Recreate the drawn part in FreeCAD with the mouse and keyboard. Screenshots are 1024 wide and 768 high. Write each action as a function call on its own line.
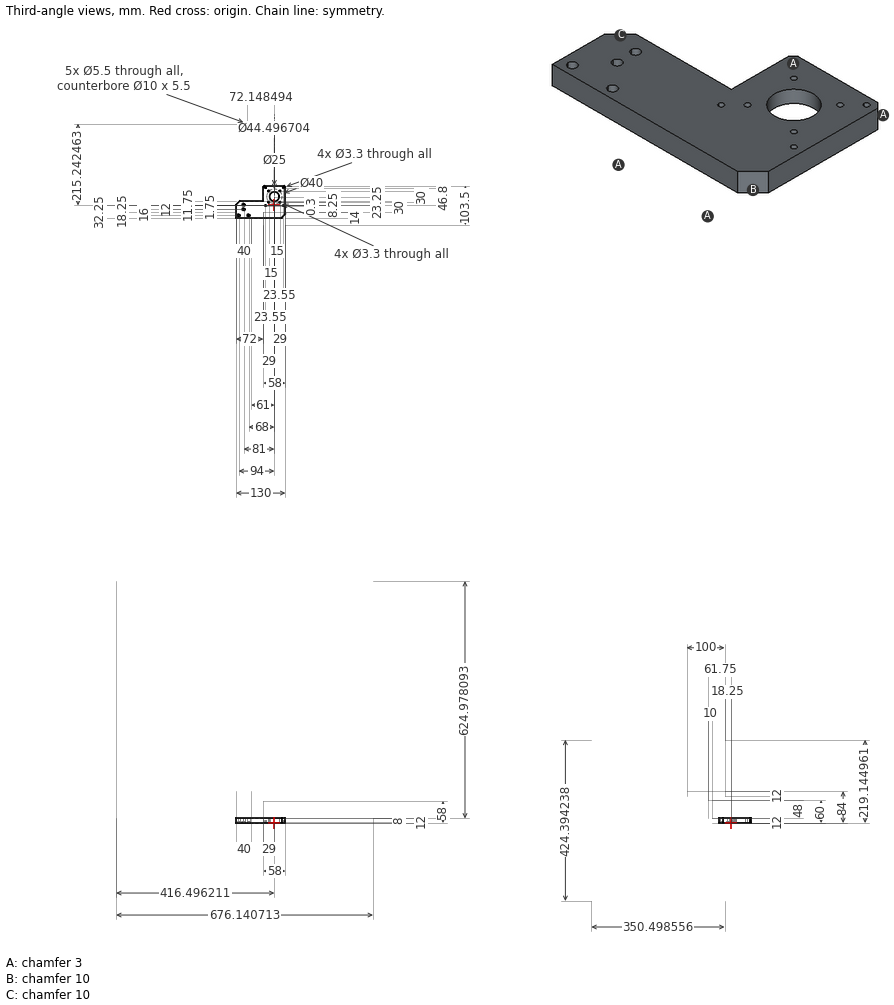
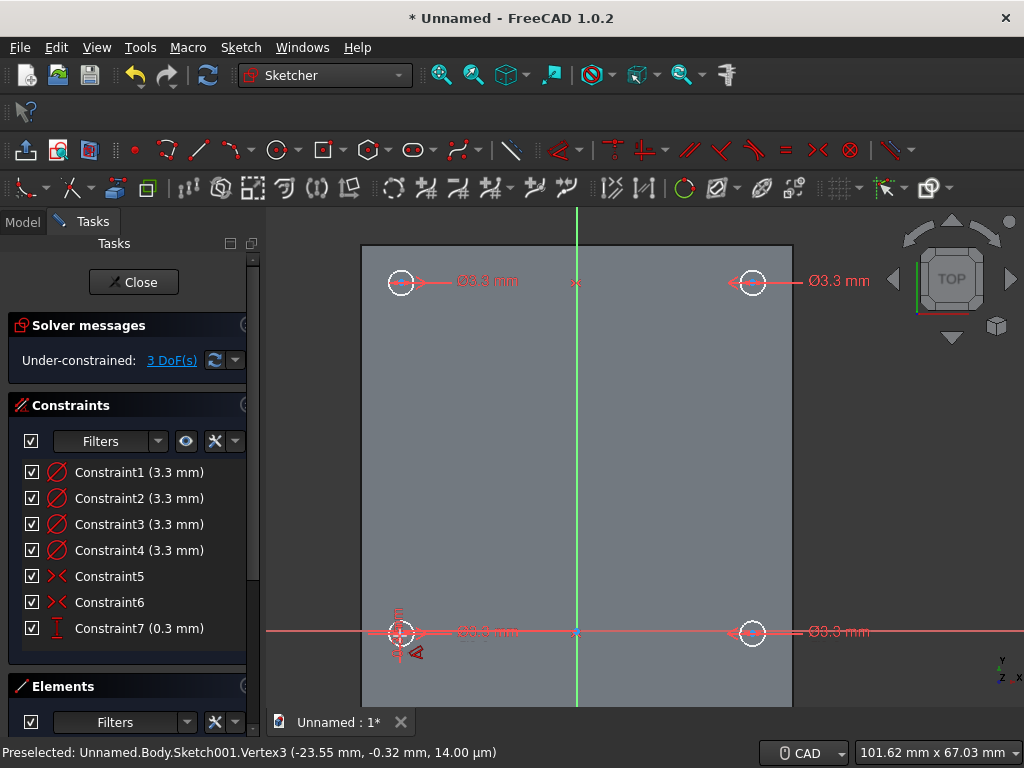
click(753, 283)
click(787, 457)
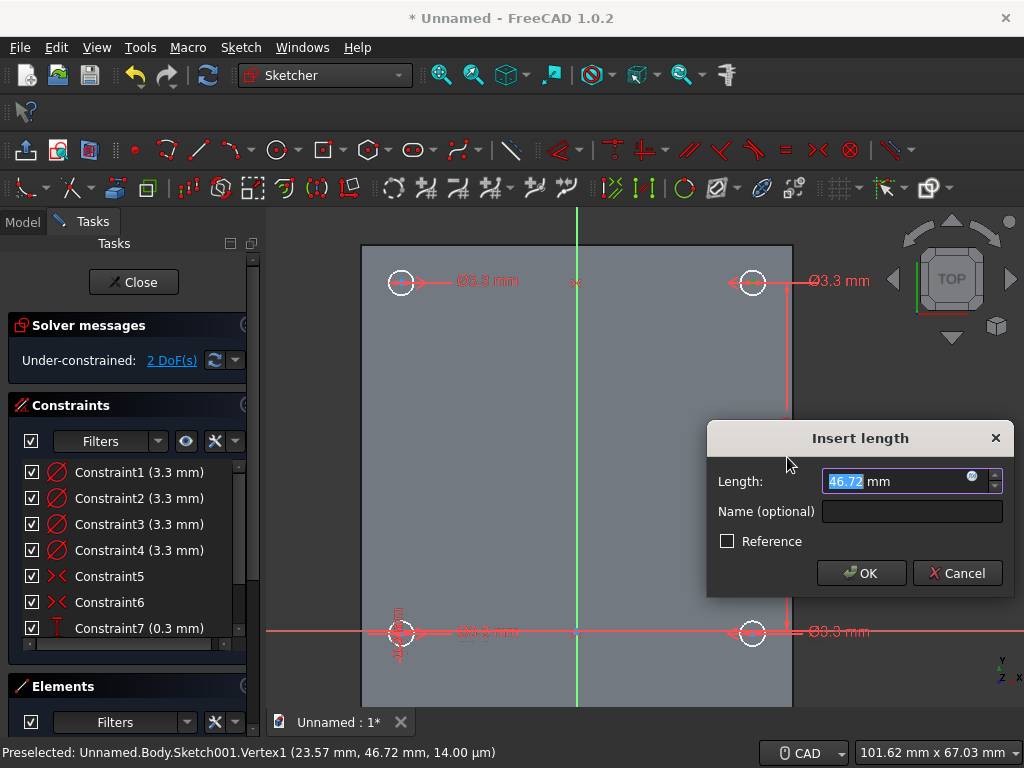
text(46.8)
key(Return)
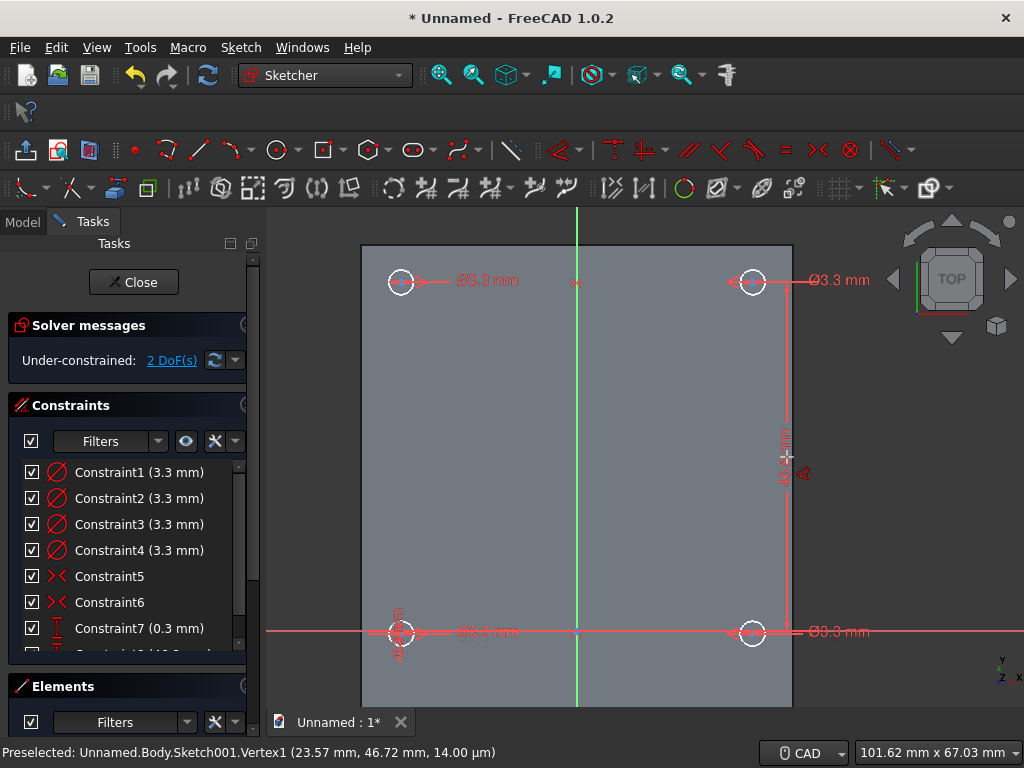
click(753, 282)
click(665, 248)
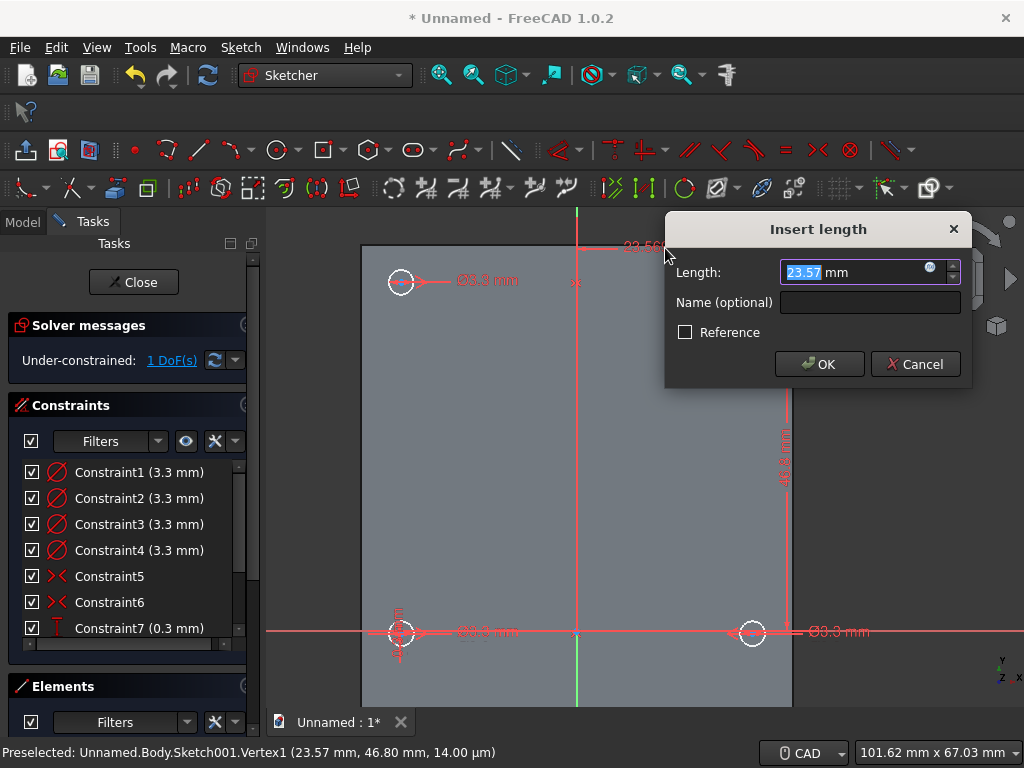
text(23.55)
key(Return)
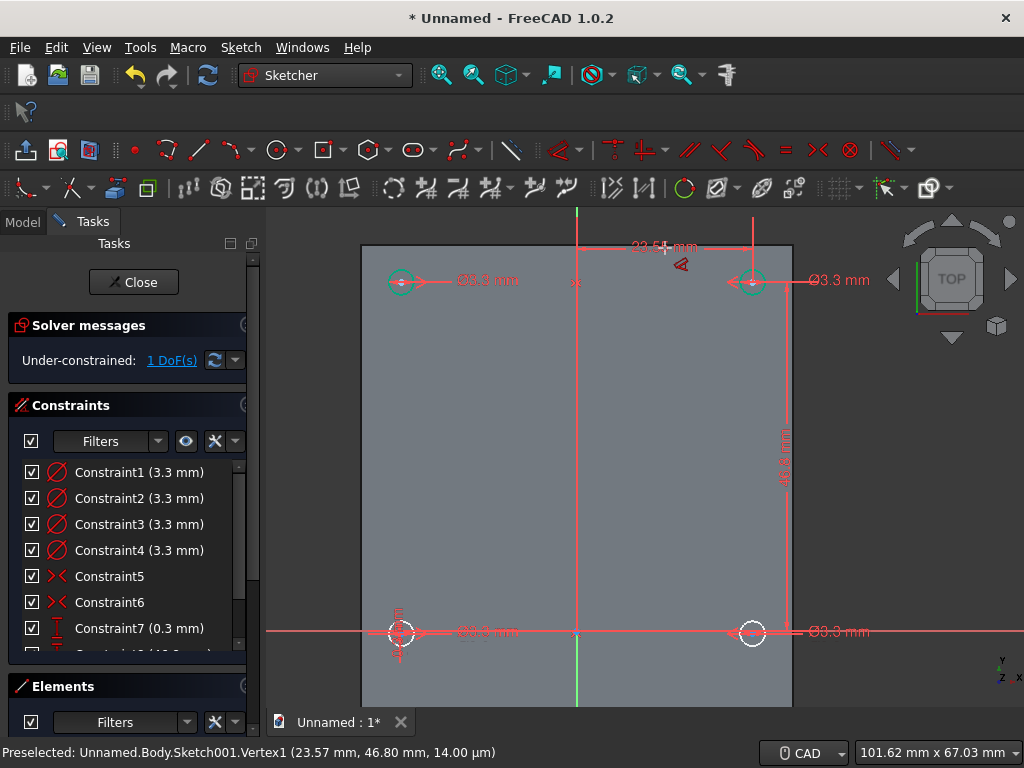
click(401, 634)
click(489, 668)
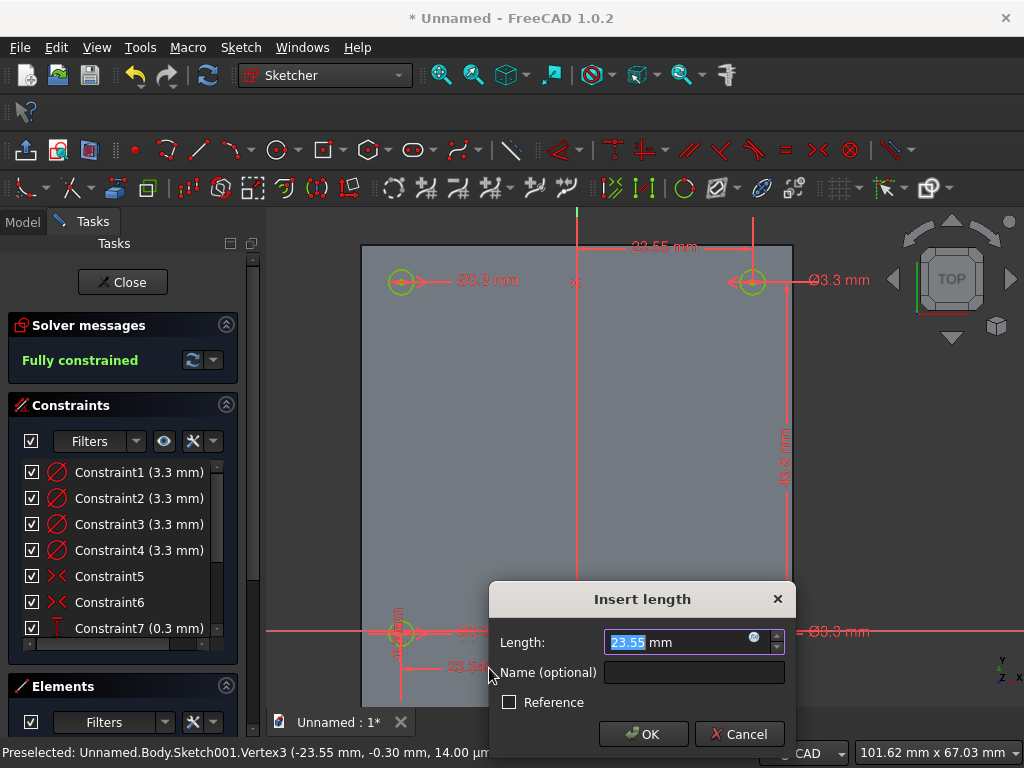
text(23.55)
key(Return)
key(Escape)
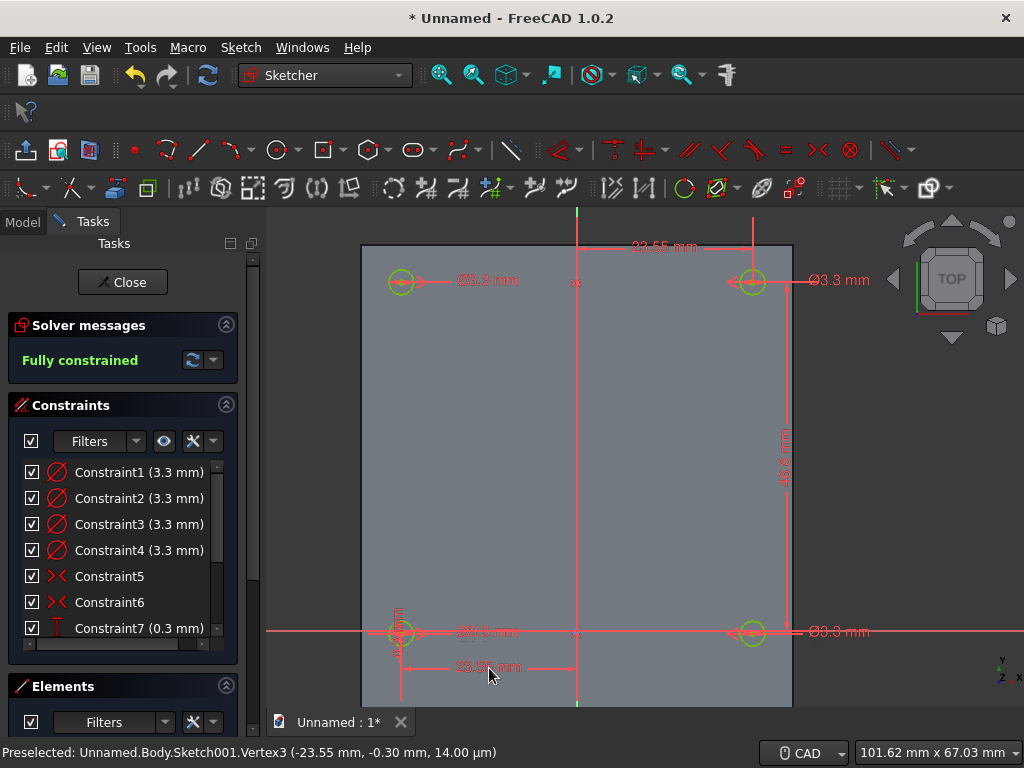
click(123, 282)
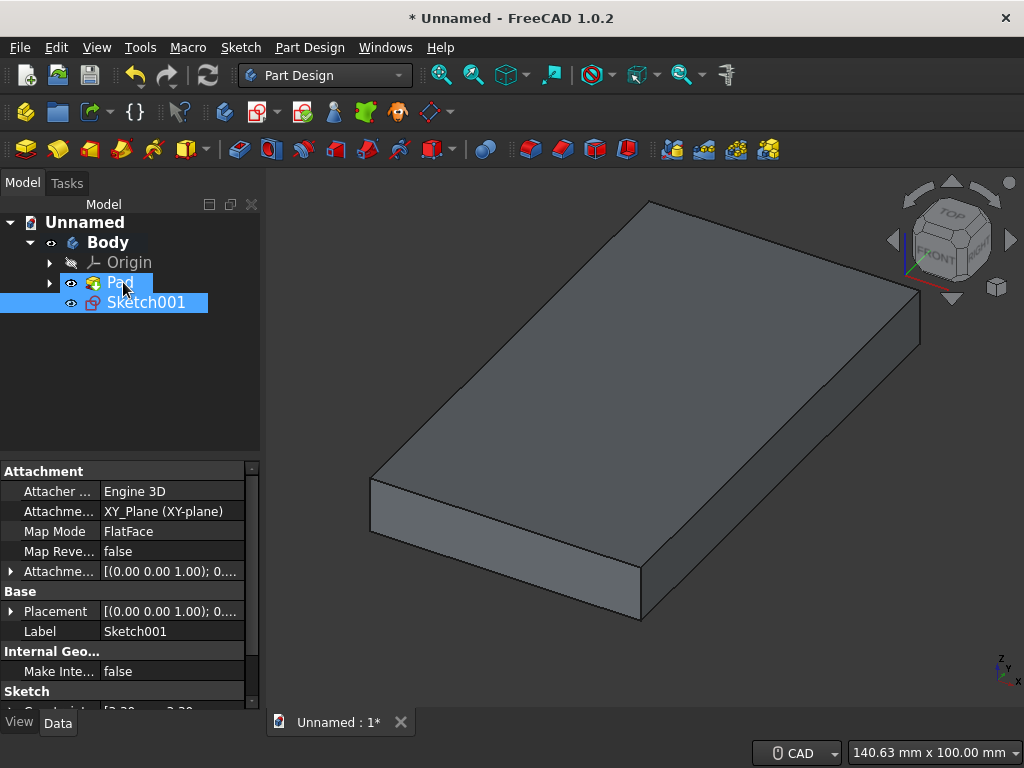
click(272, 150)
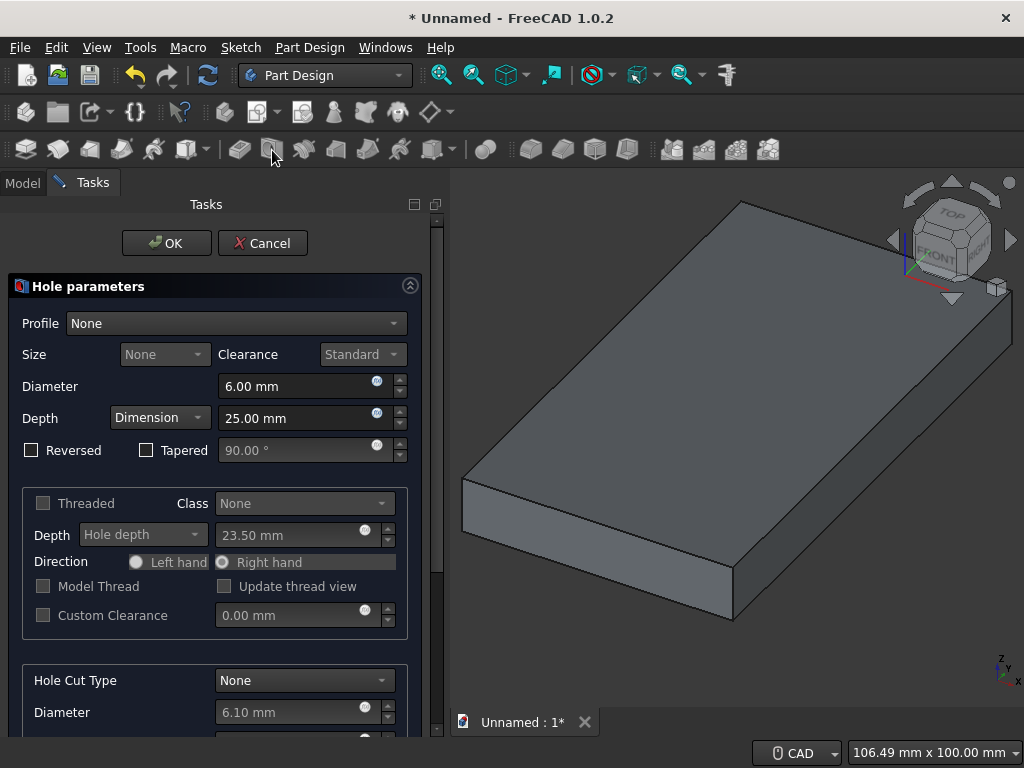
triple_click(305, 386)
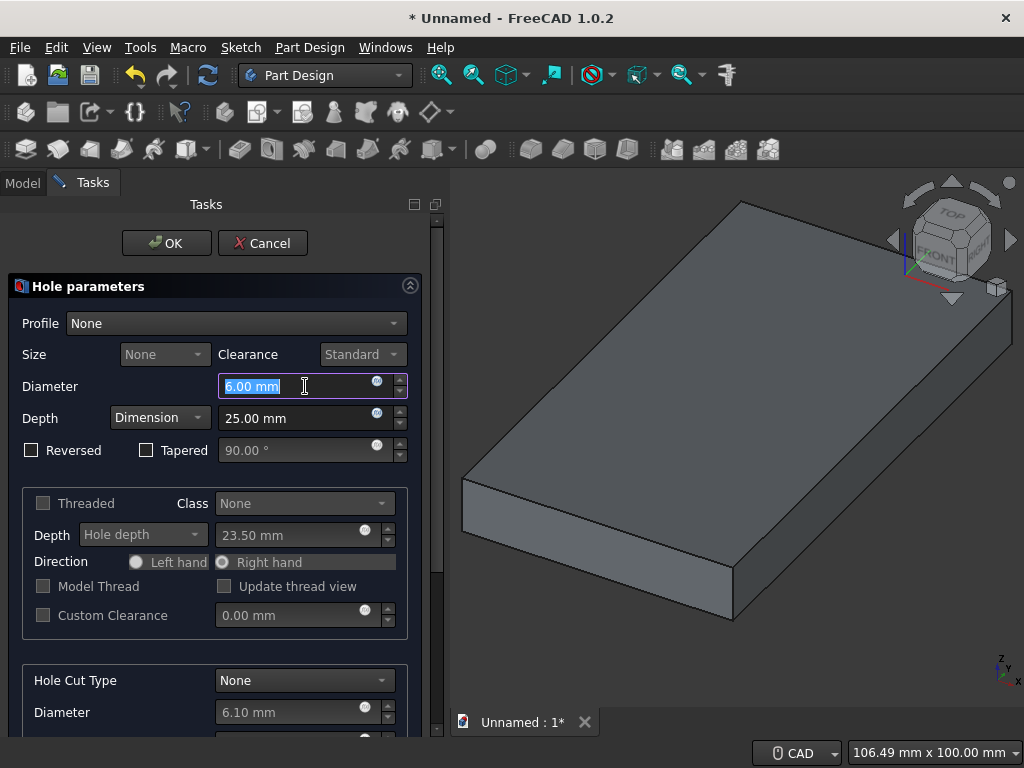
text(3.3)
key(Tab)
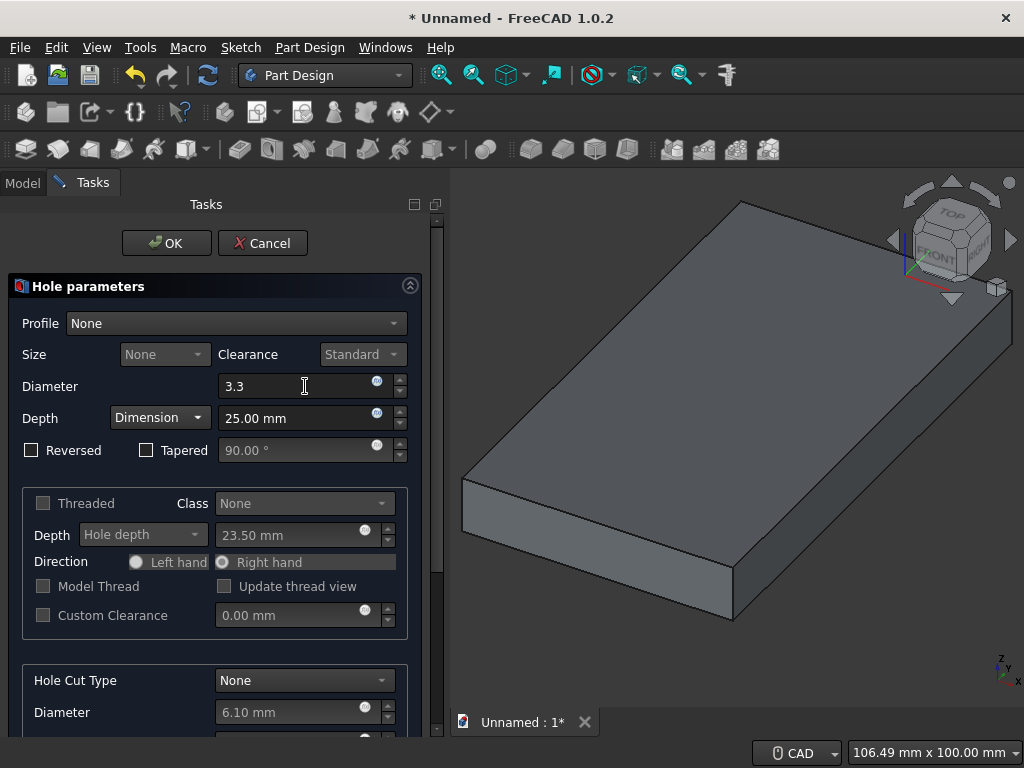
click(161, 418)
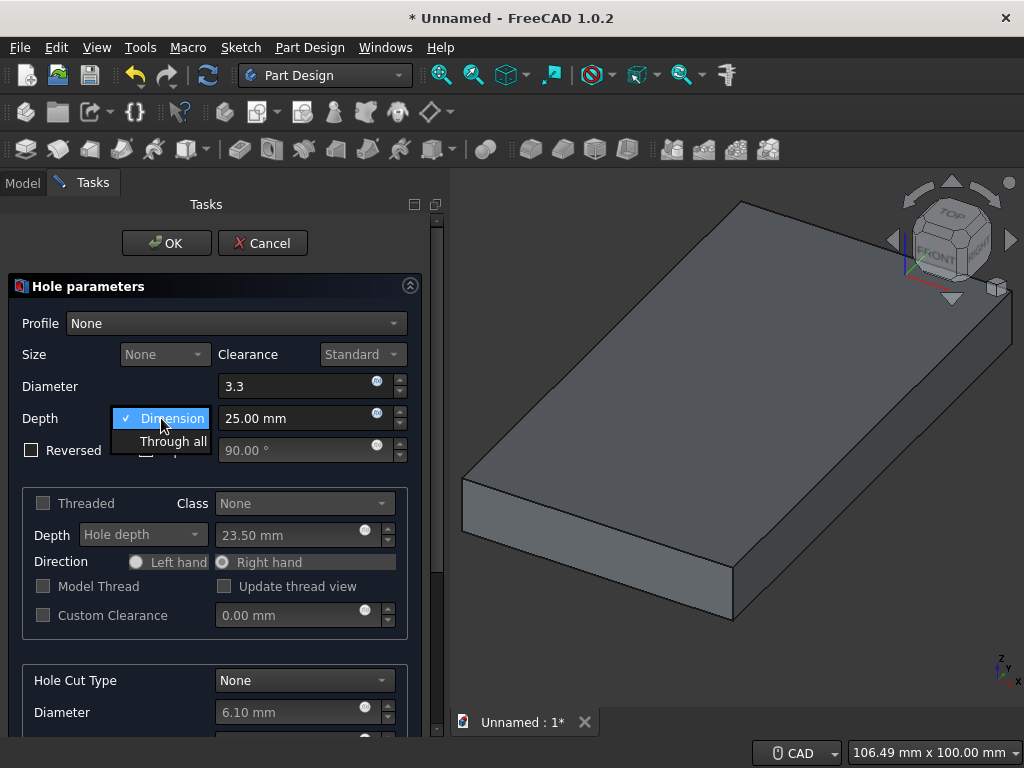
click(160, 442)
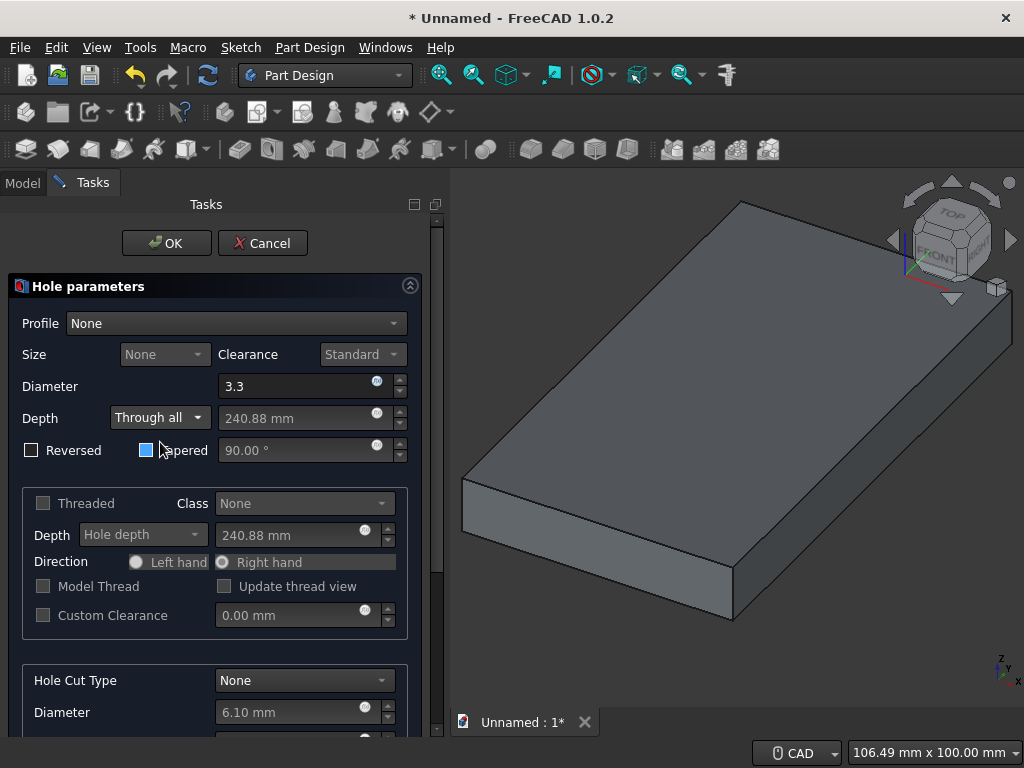
click(30, 450)